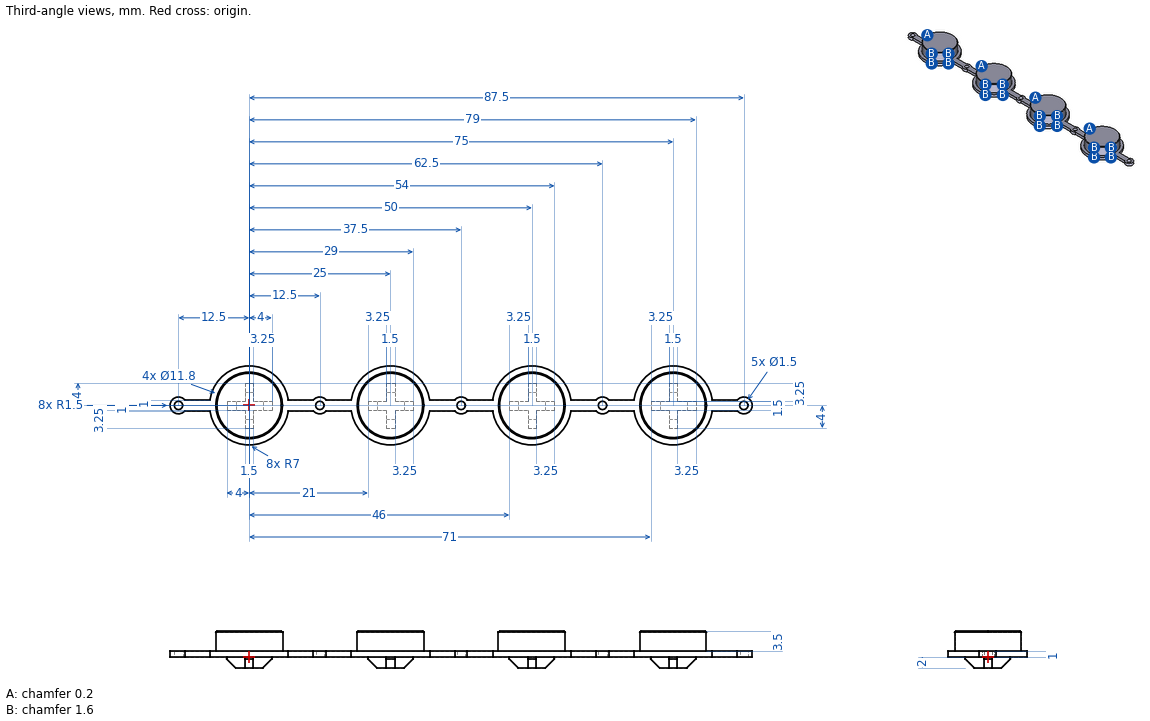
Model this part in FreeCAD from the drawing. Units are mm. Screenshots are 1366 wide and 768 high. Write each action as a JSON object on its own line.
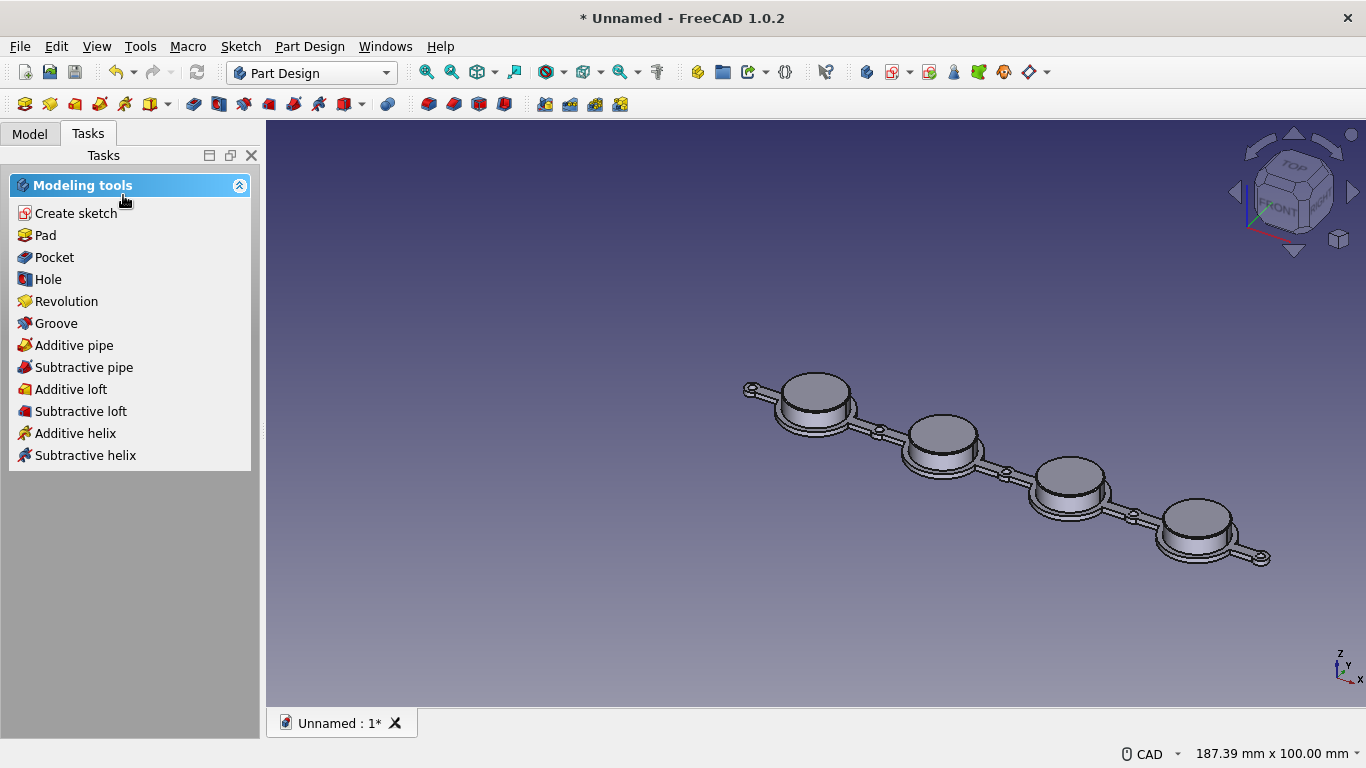
{"action": "left_click", "coordinate": [25, 104]}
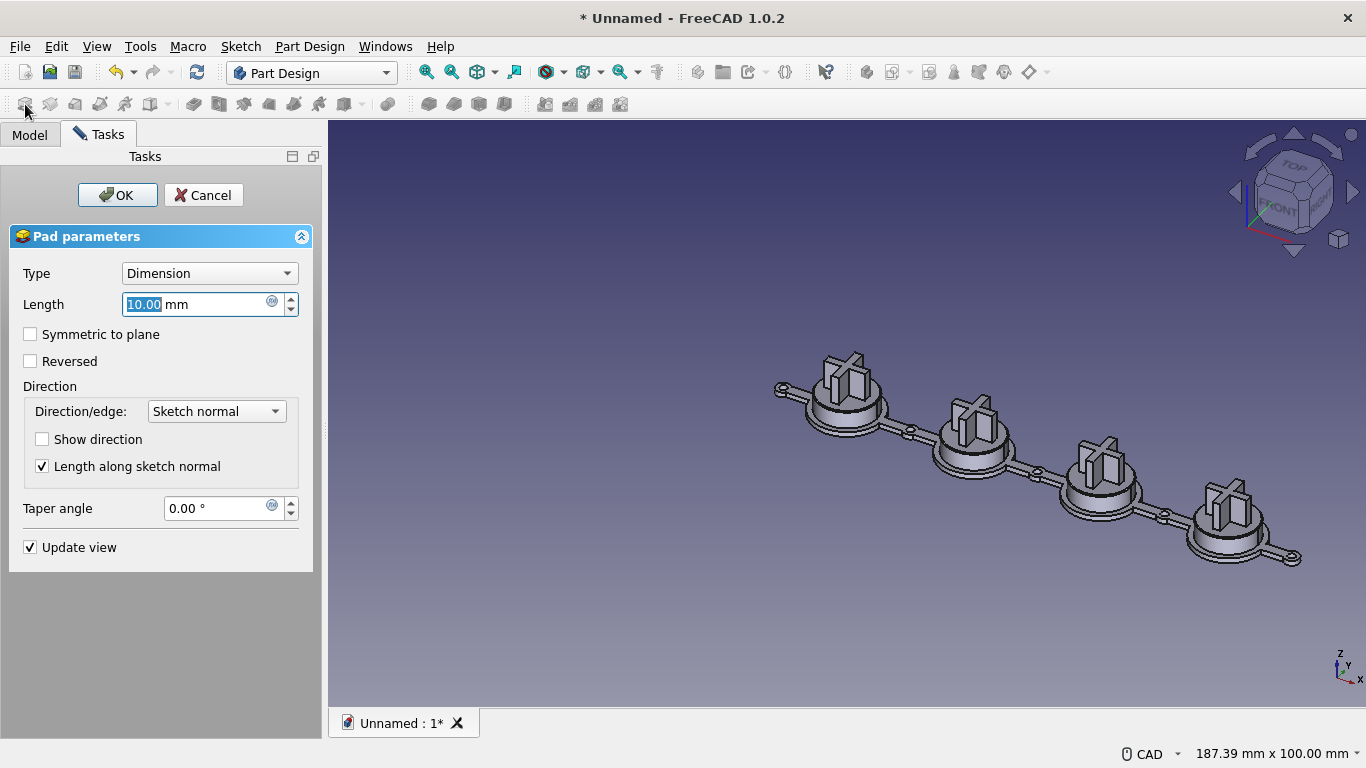
{"action": "type", "text": "2"}
{"action": "key", "text": "Tab"}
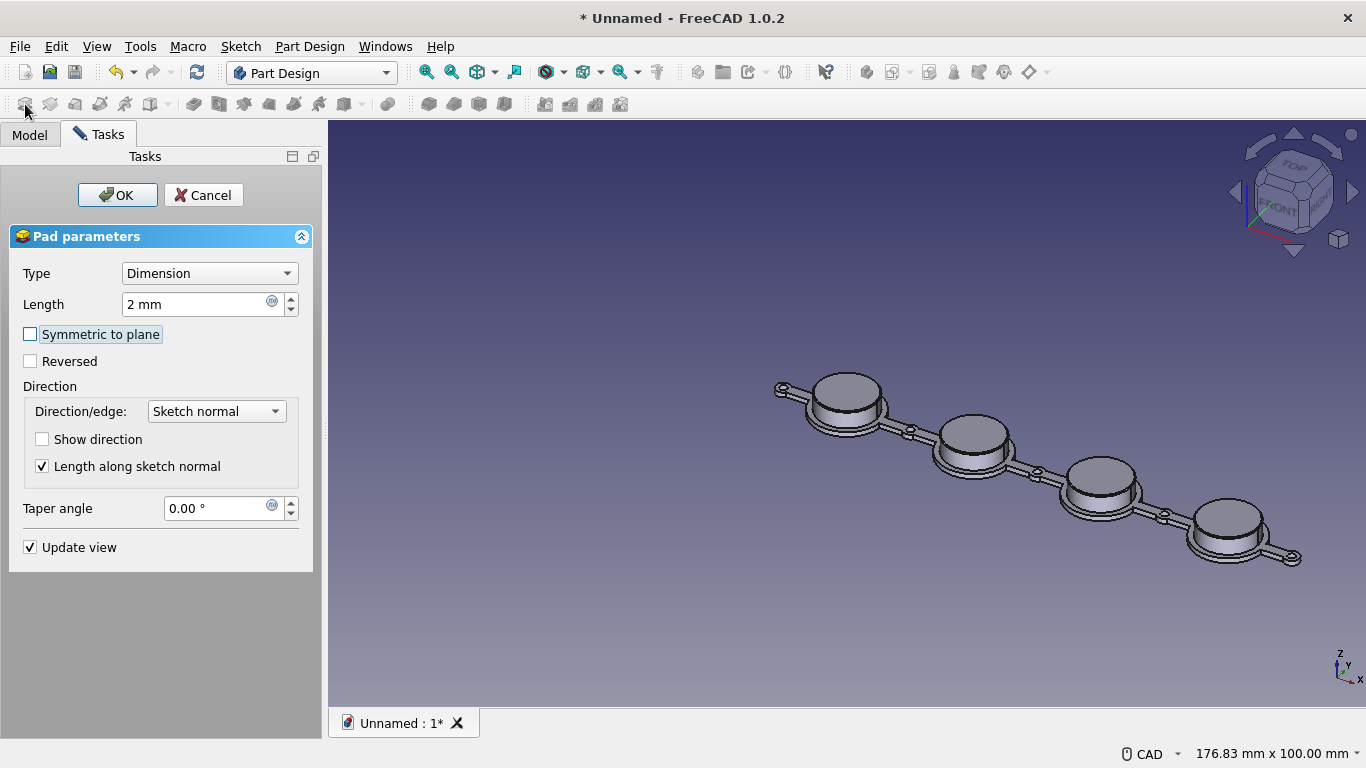
{"action": "left_click", "coordinate": [31, 361]}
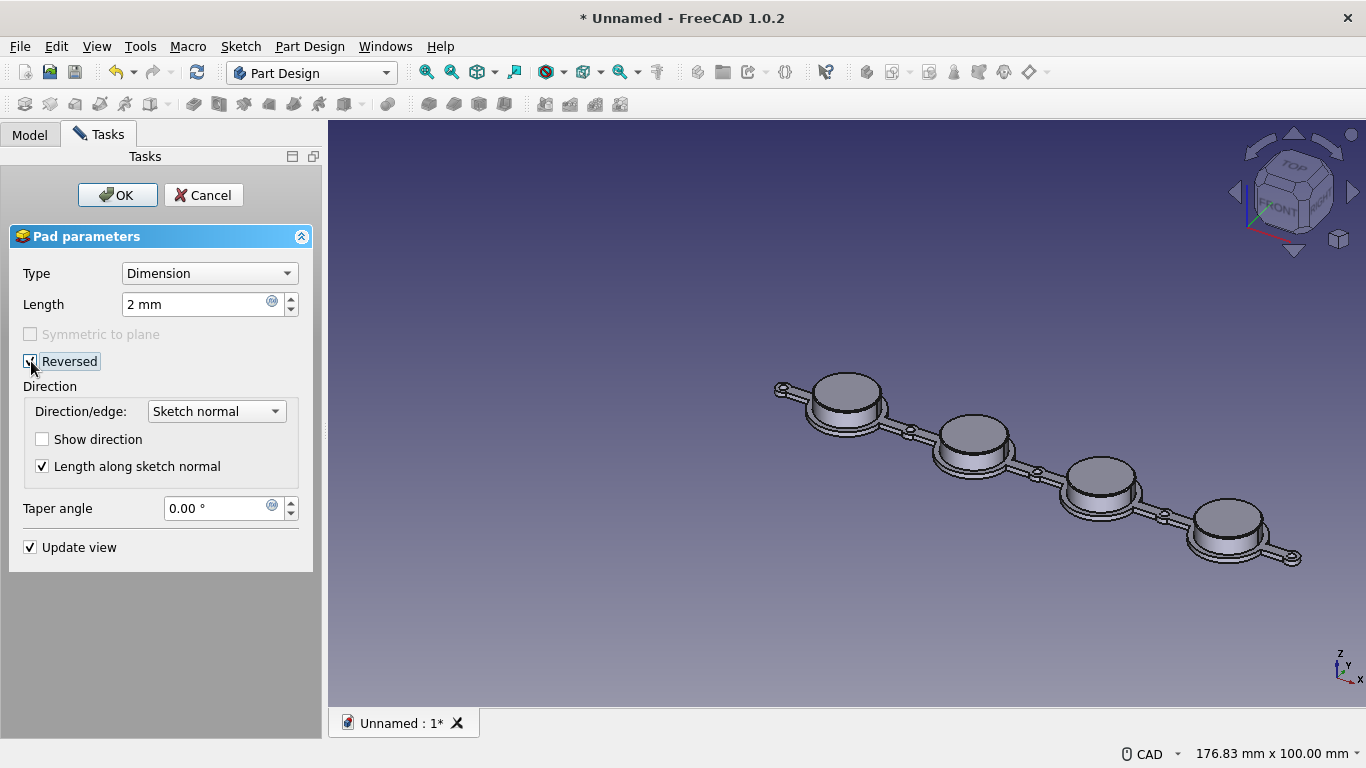
{"action": "left_click", "coordinate": [118, 195]}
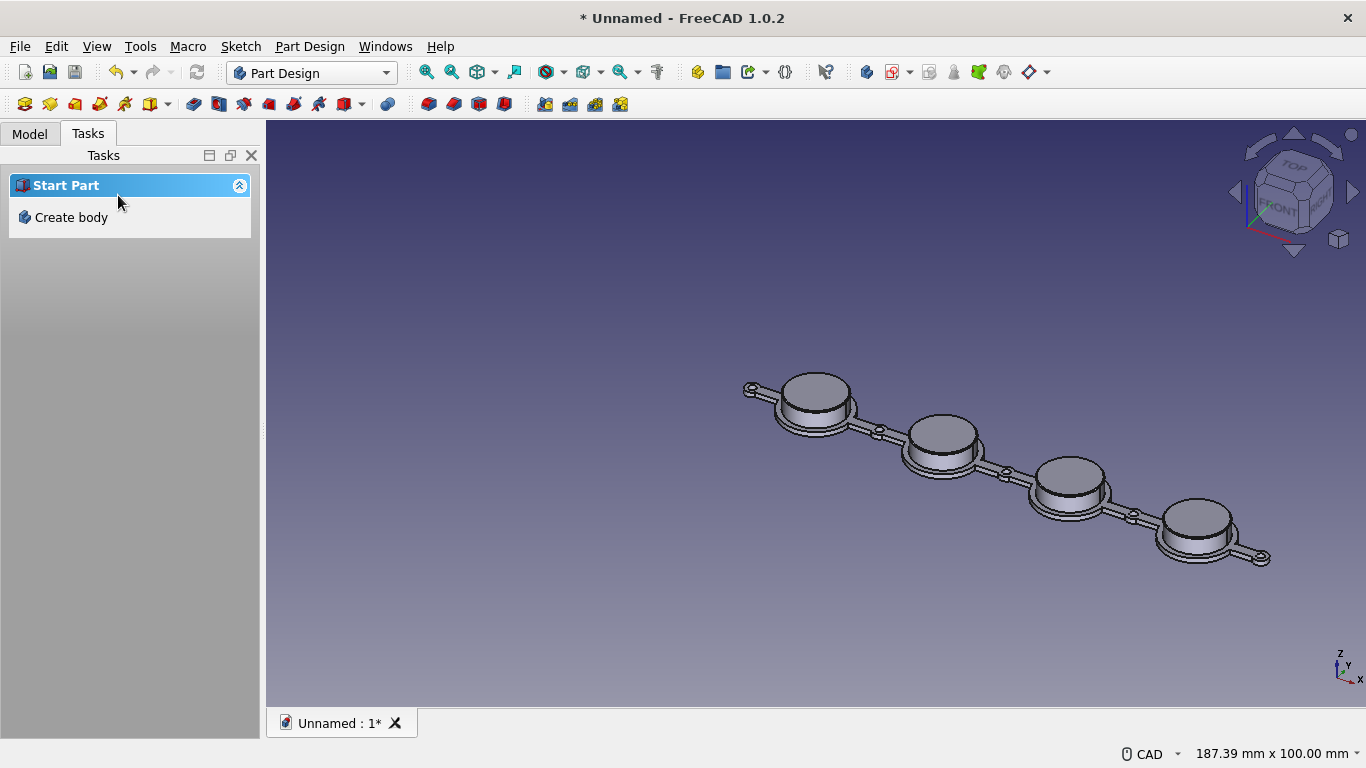
{"action": "scroll", "coordinate": [1186, 560], "scroll_direction": "up", "scroll_amount": 8}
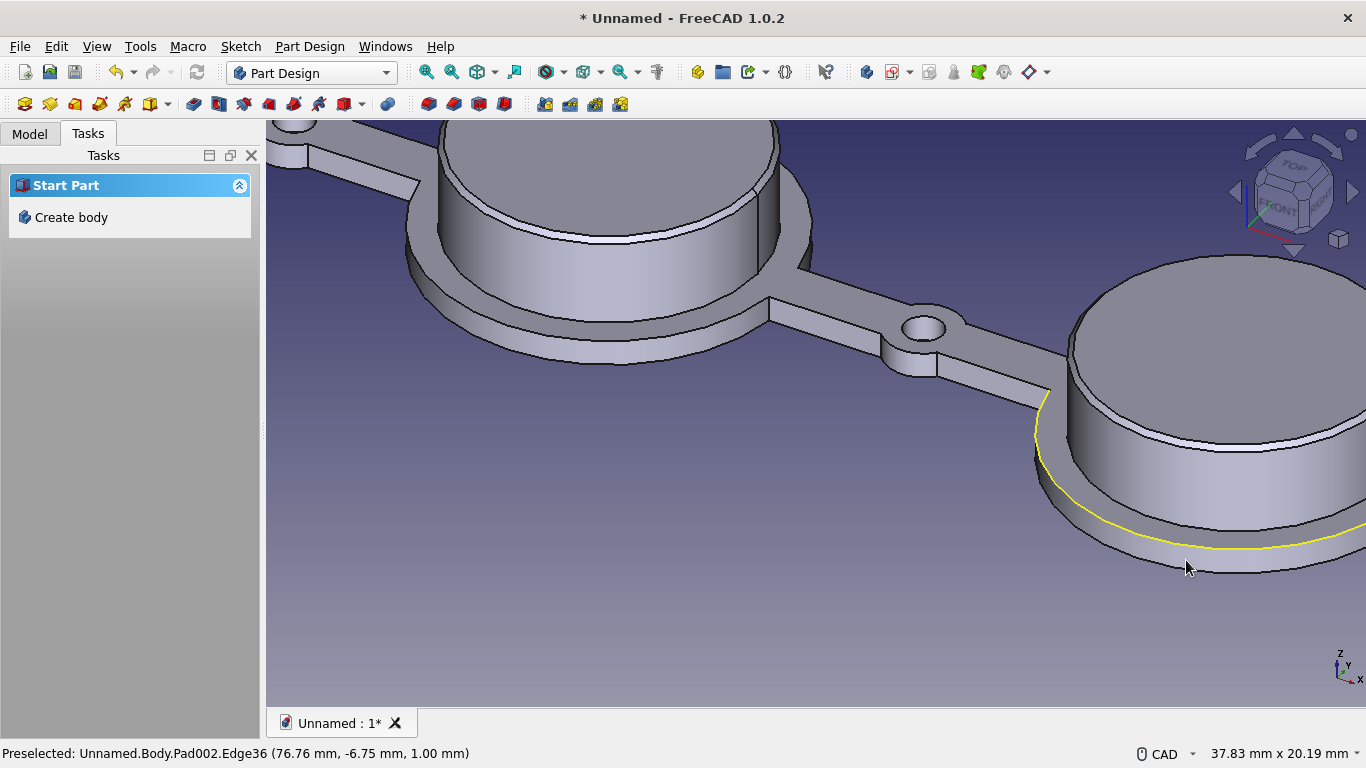
{"action": "left_click", "coordinate": [427, 72]}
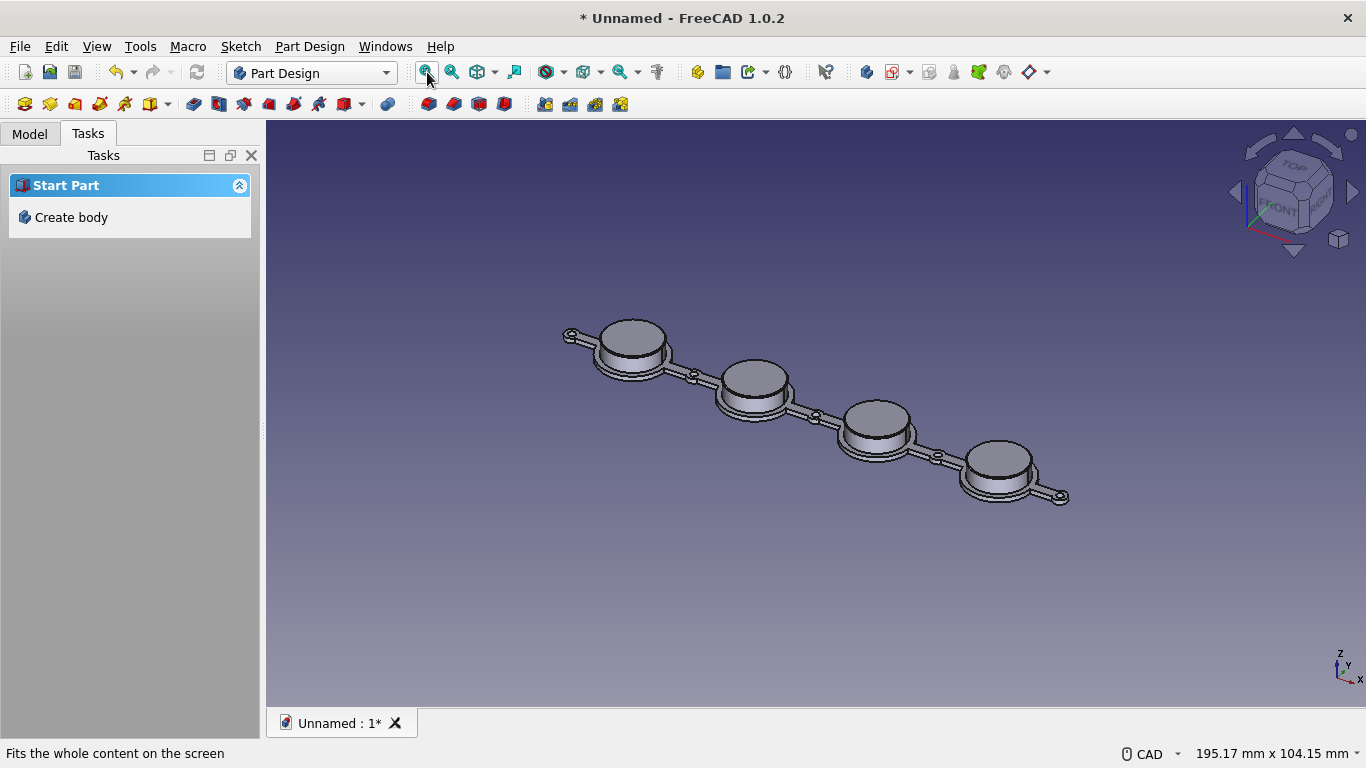
{"action": "key", "text": "0"}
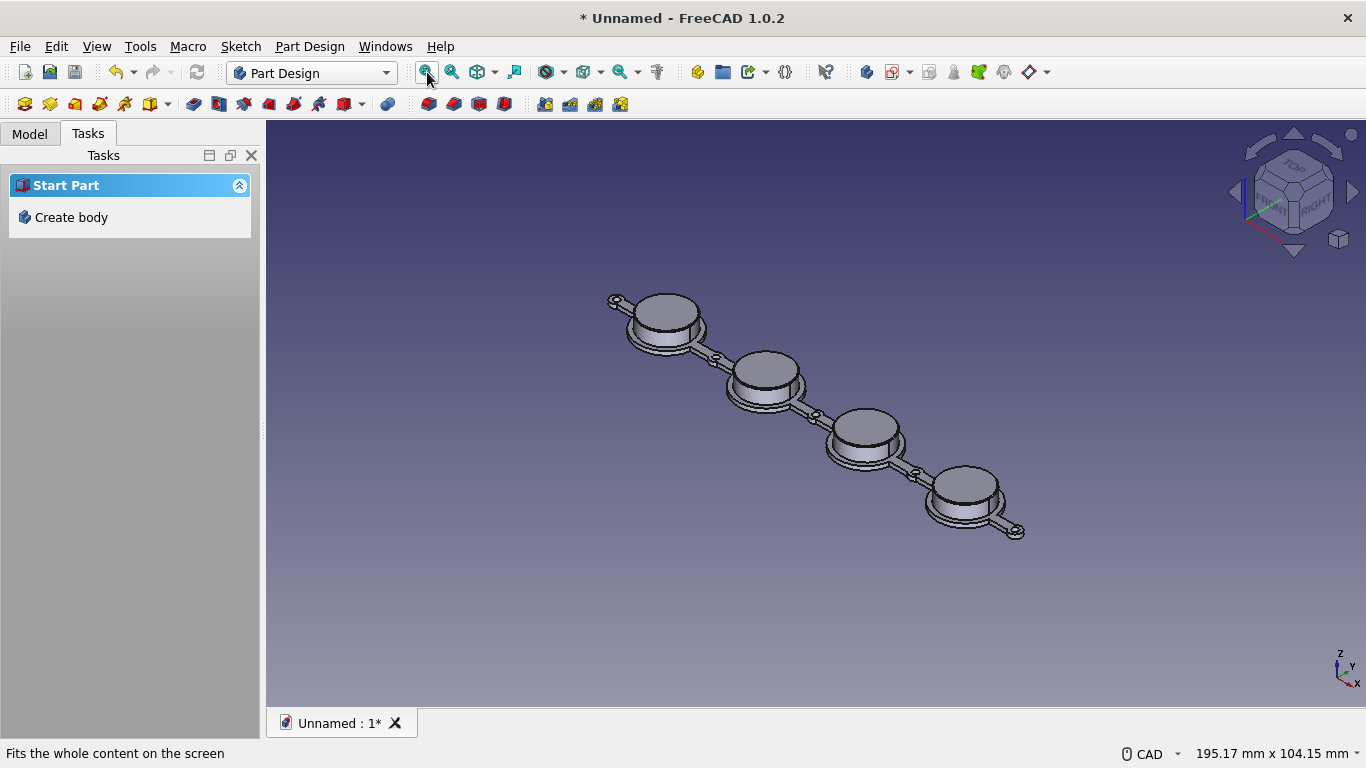
{"action": "scroll", "coordinate": [950, 523], "scroll_direction": "up", "scroll_amount": 8}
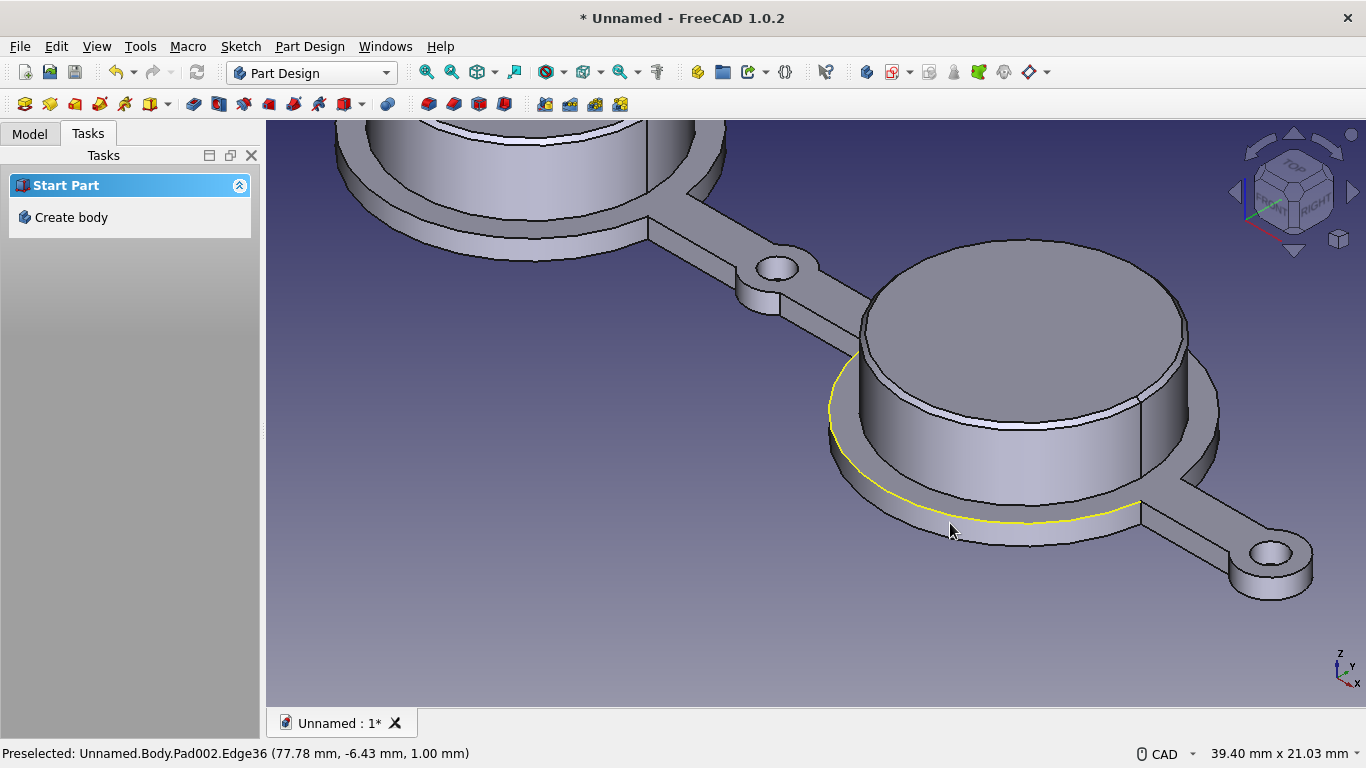
{"action": "key", "text": "v f"}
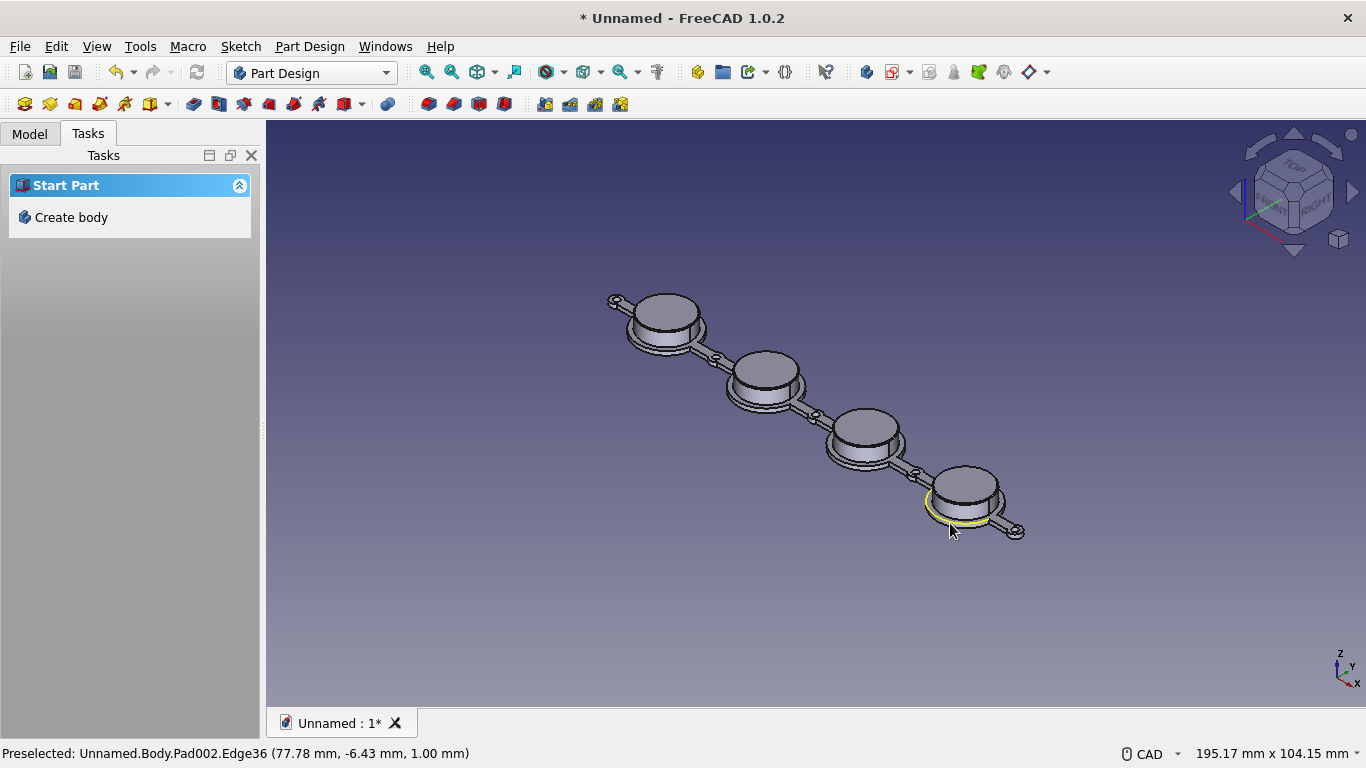
{"action": "key", "text": "2"}